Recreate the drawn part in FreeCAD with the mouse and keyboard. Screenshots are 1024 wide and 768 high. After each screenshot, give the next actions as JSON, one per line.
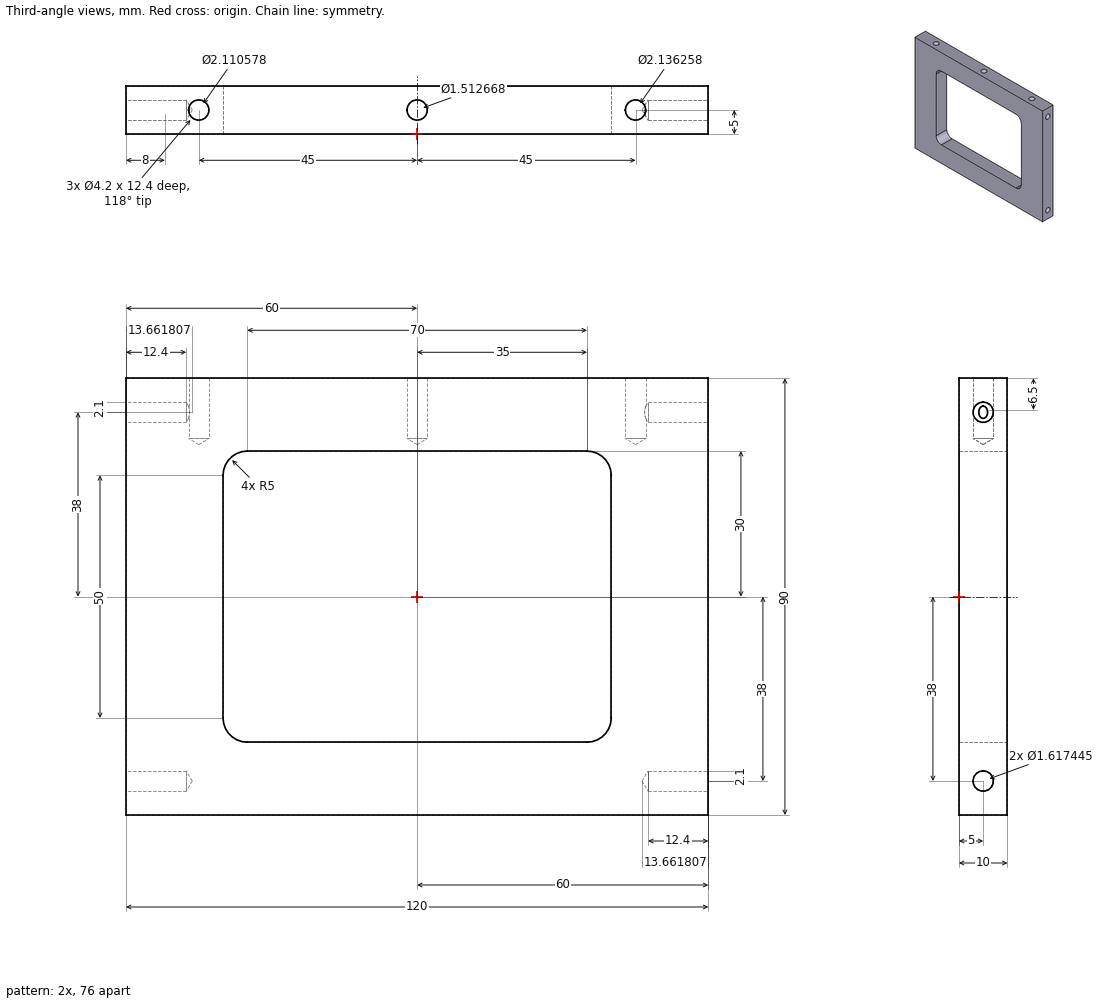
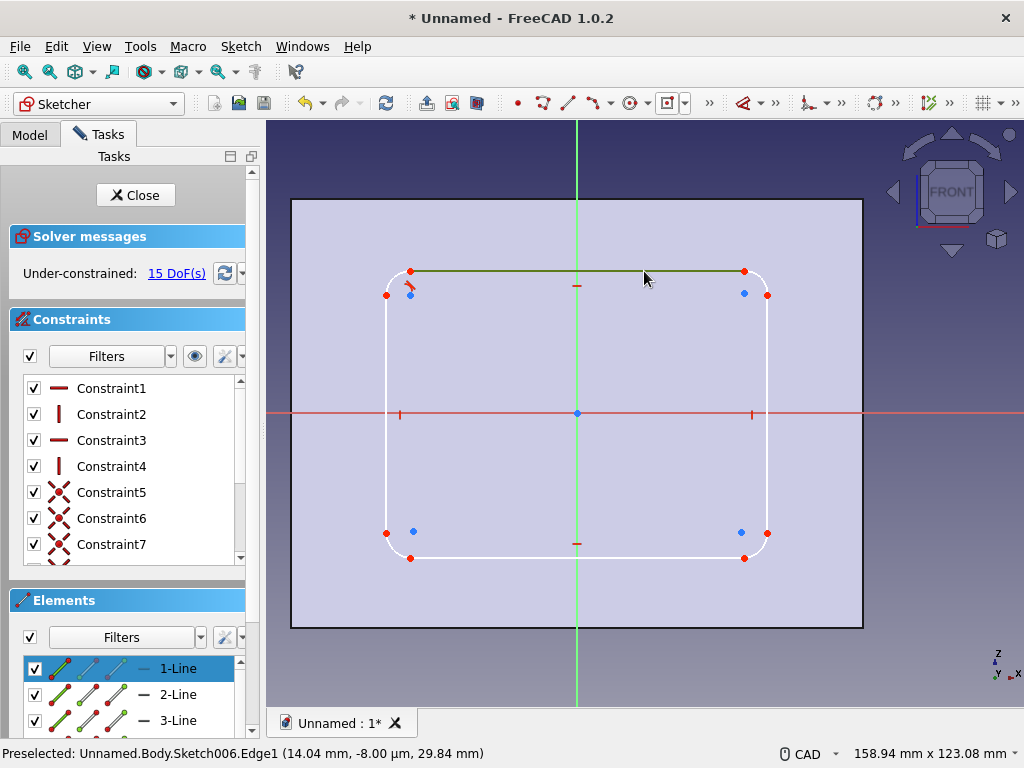
{"action": "left_click", "coordinate": [765, 284]}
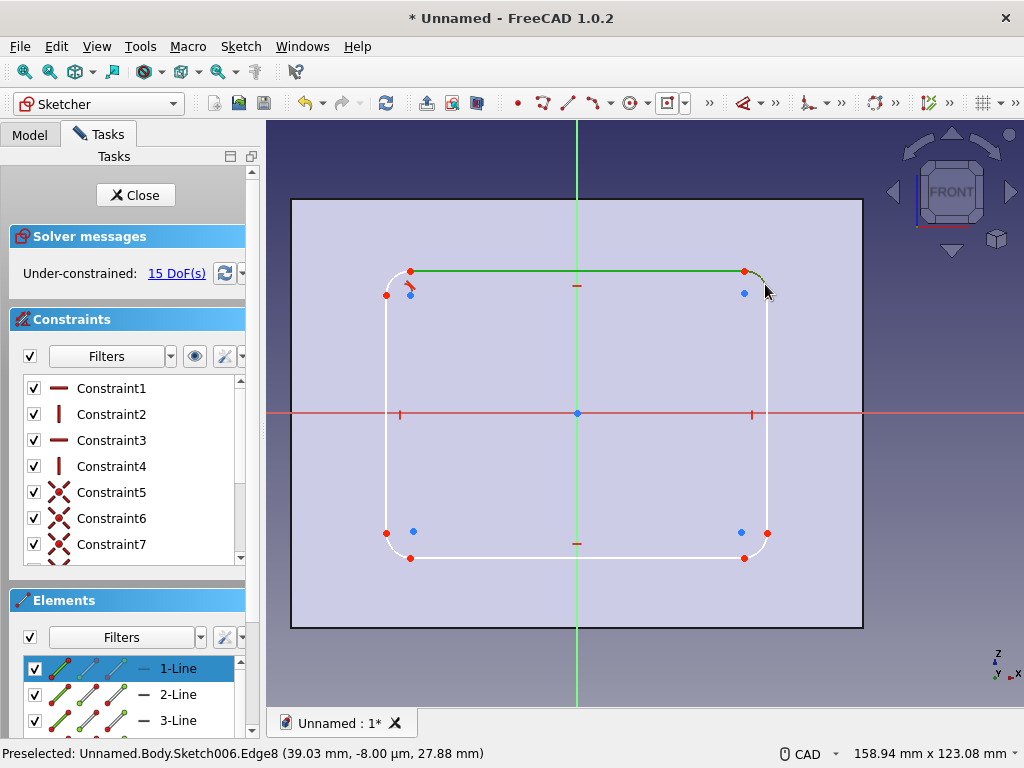
{"action": "key", "text": "t"}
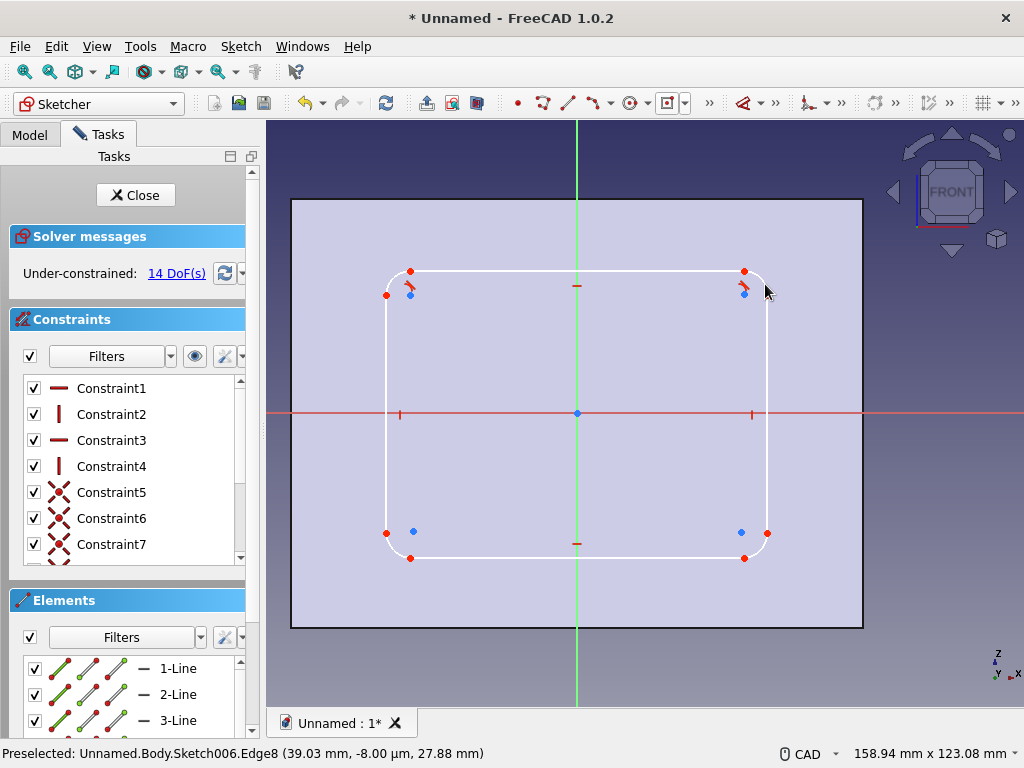
{"action": "left_click", "coordinate": [386, 367]}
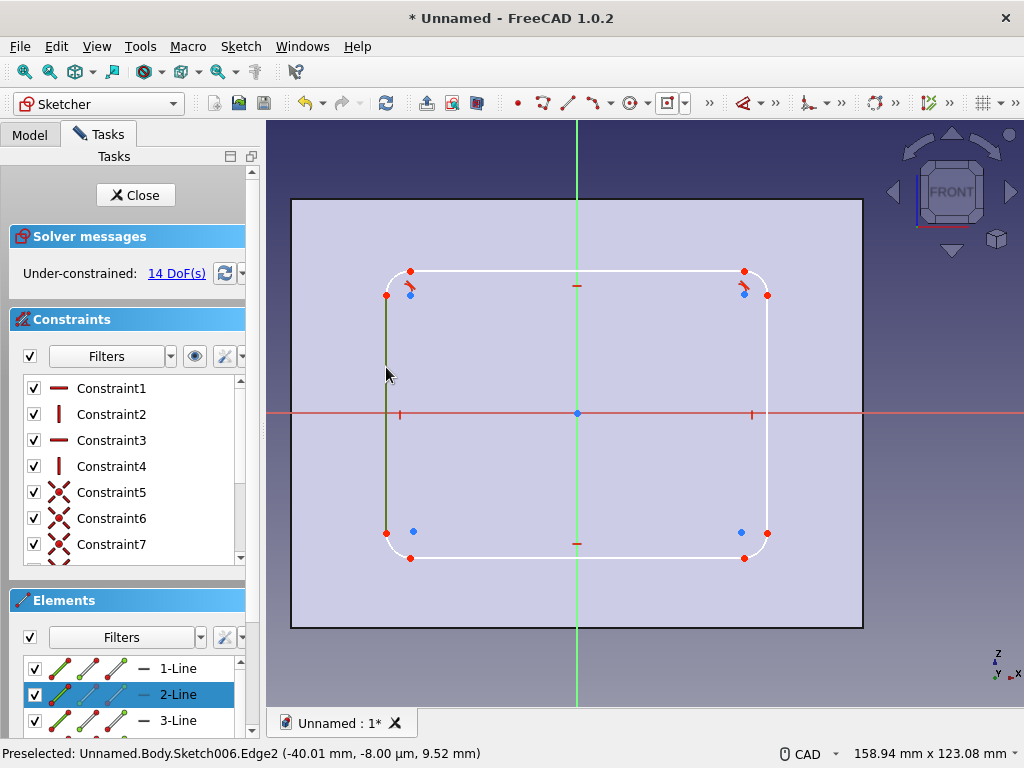
{"action": "left_click", "coordinate": [400, 274]}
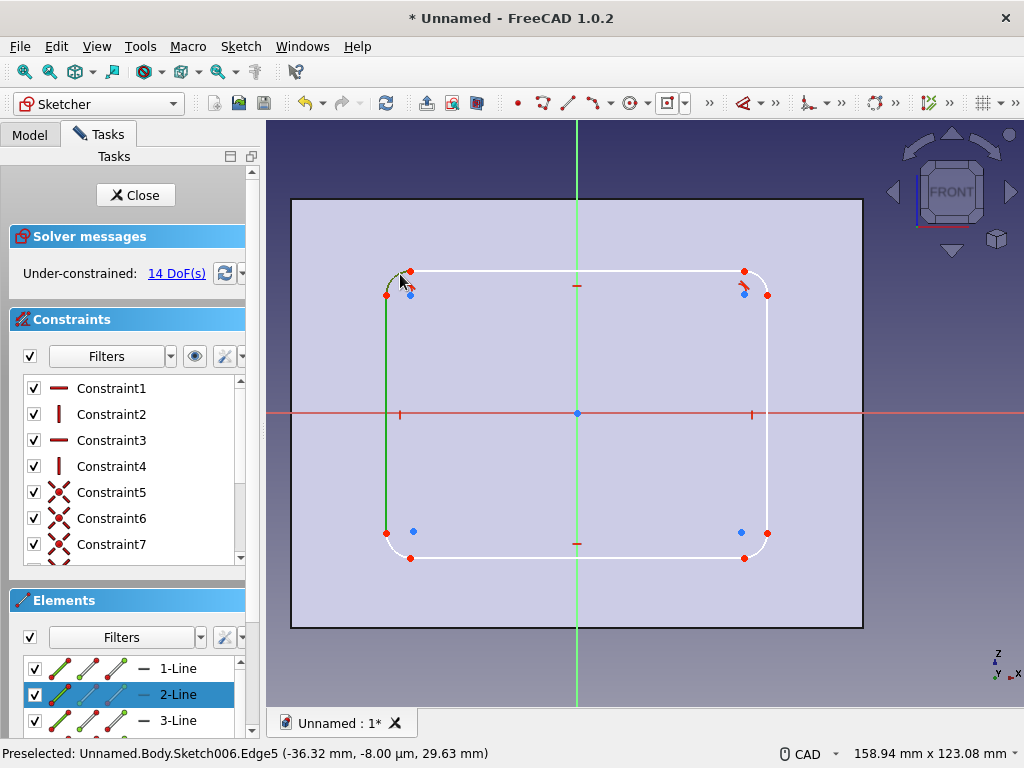
{"action": "key", "text": "t"}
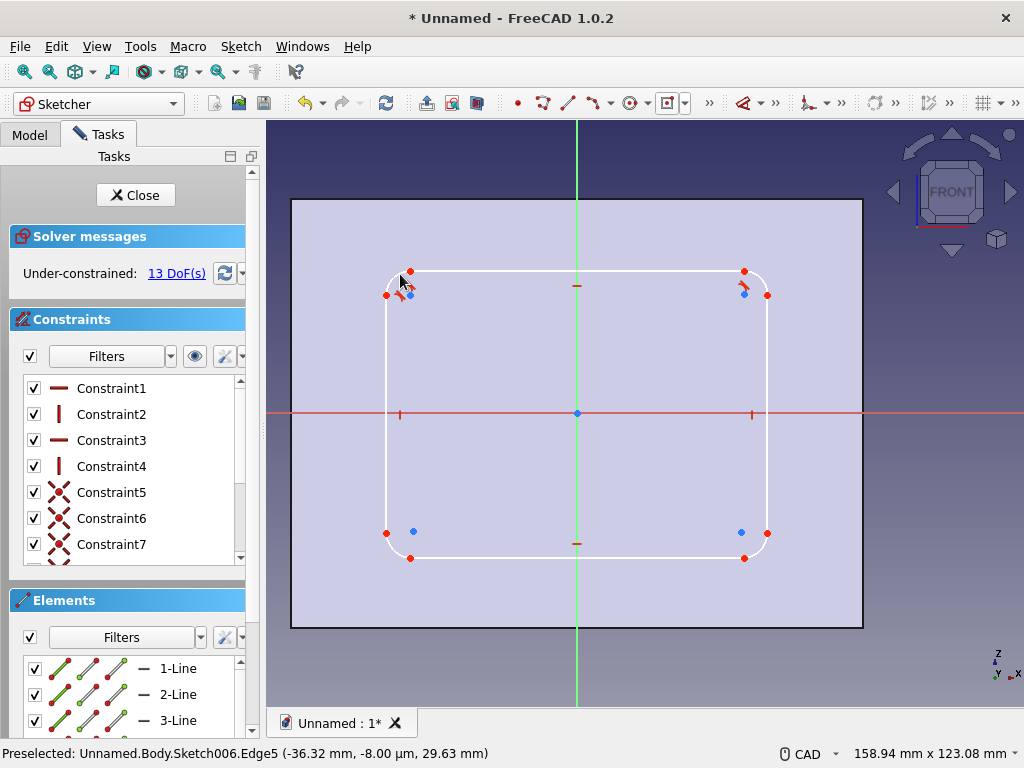
{"action": "left_click", "coordinate": [386, 367]}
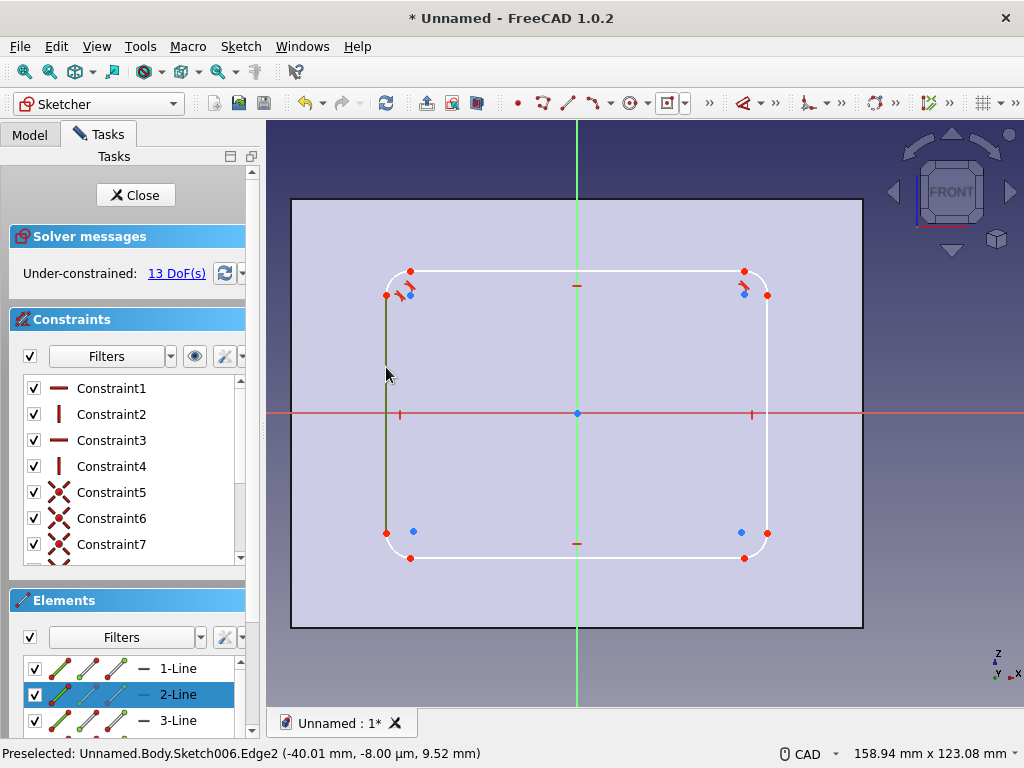
{"action": "scroll", "coordinate": [390, 544], "scroll_direction": "up", "scroll_amount": 2}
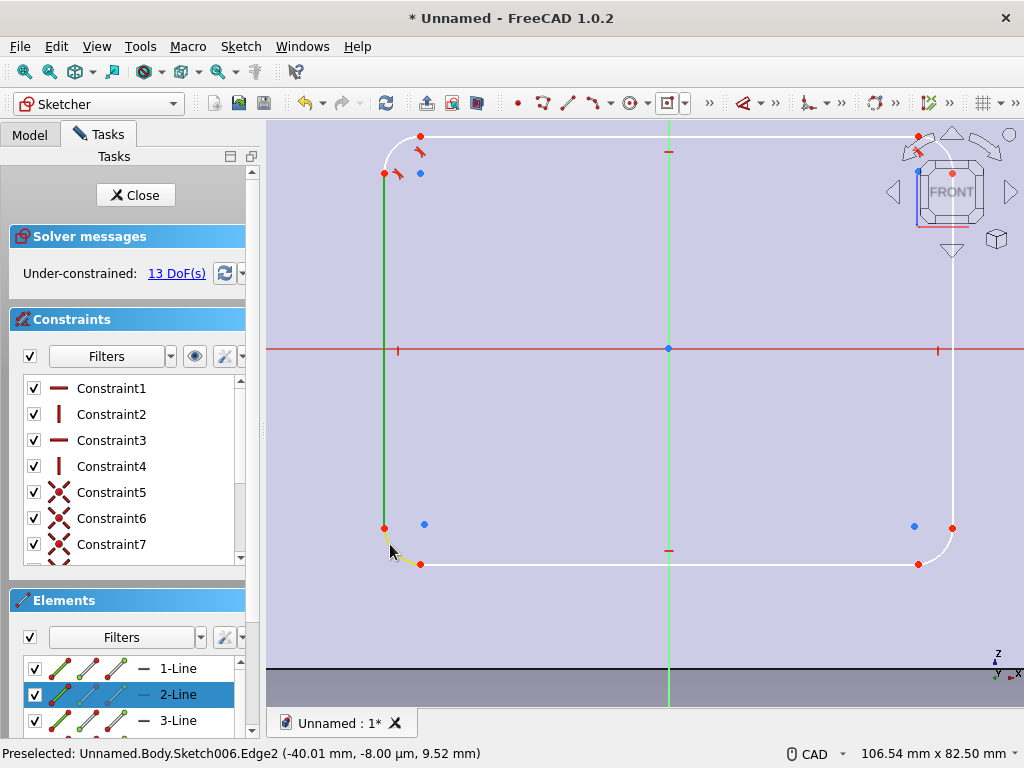
{"action": "left_click", "coordinate": [389, 544]}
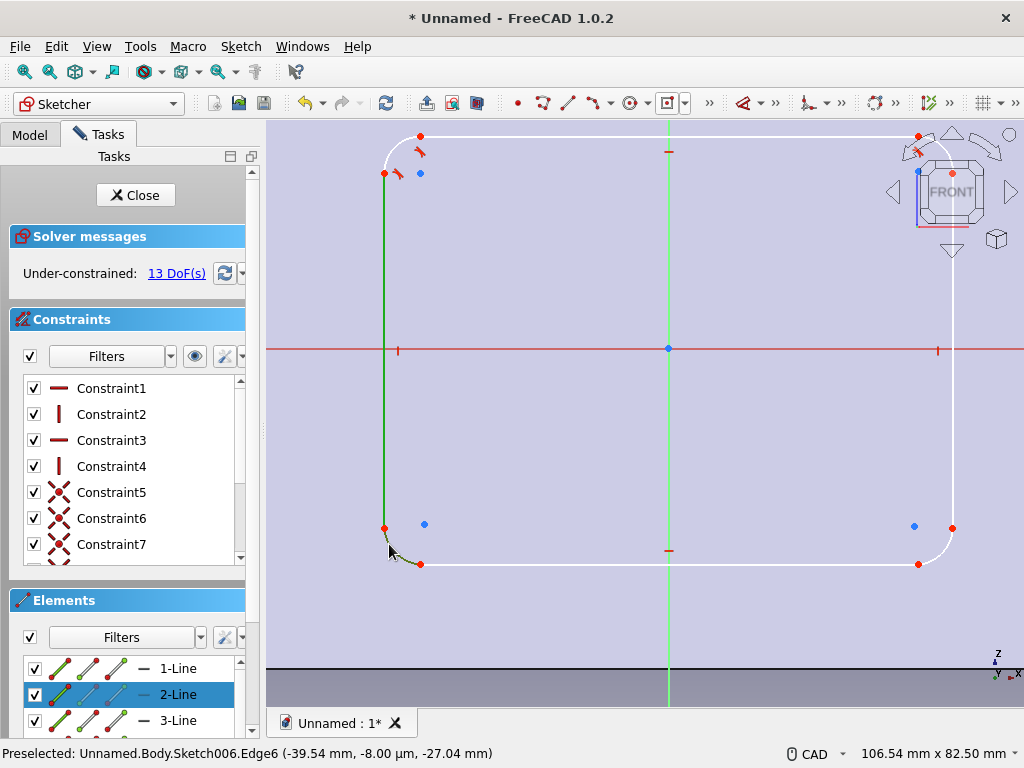
{"action": "key", "text": "t"}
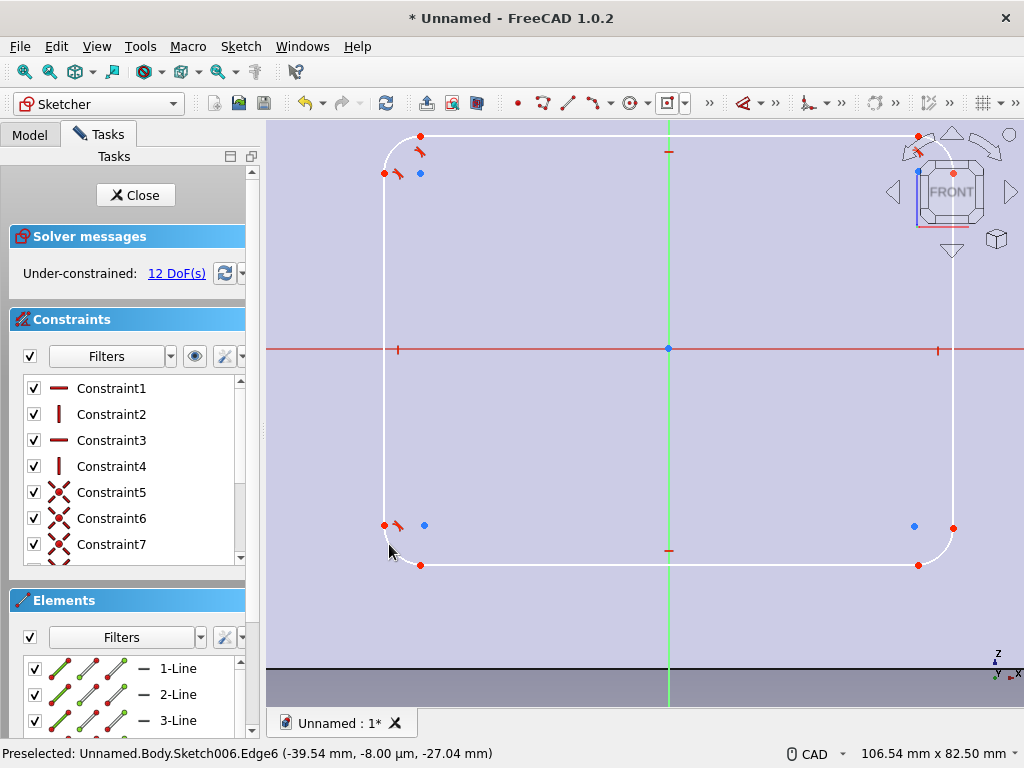
{"action": "left_click", "coordinate": [570, 565]}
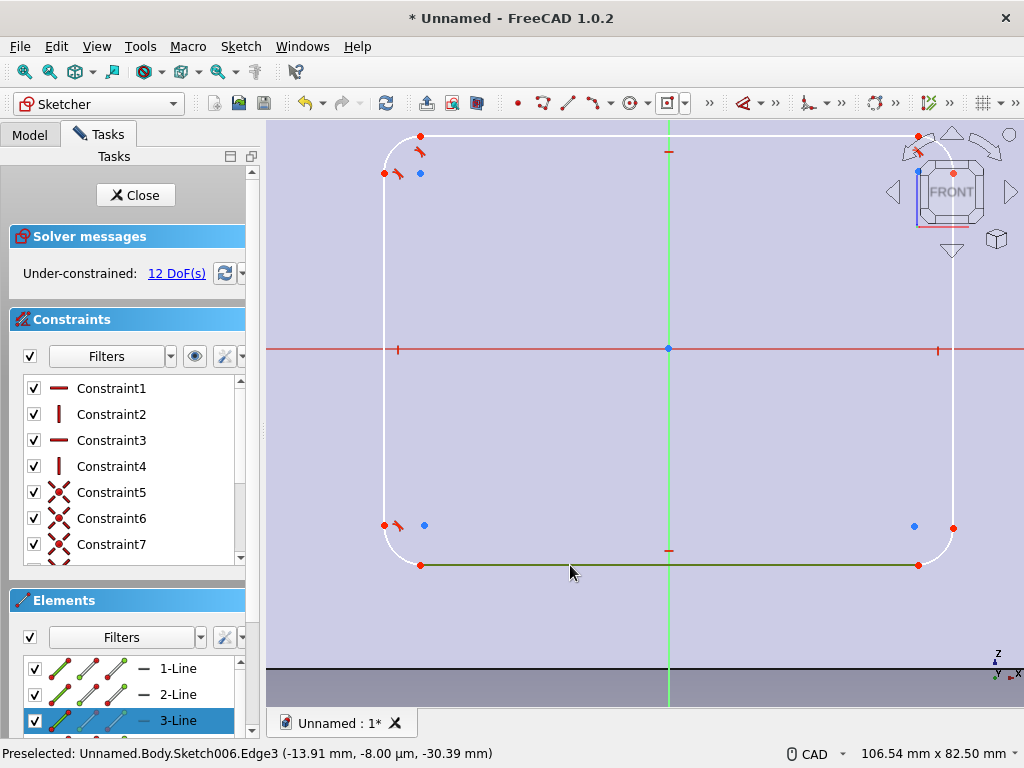
{"action": "left_click", "coordinate": [388, 542]}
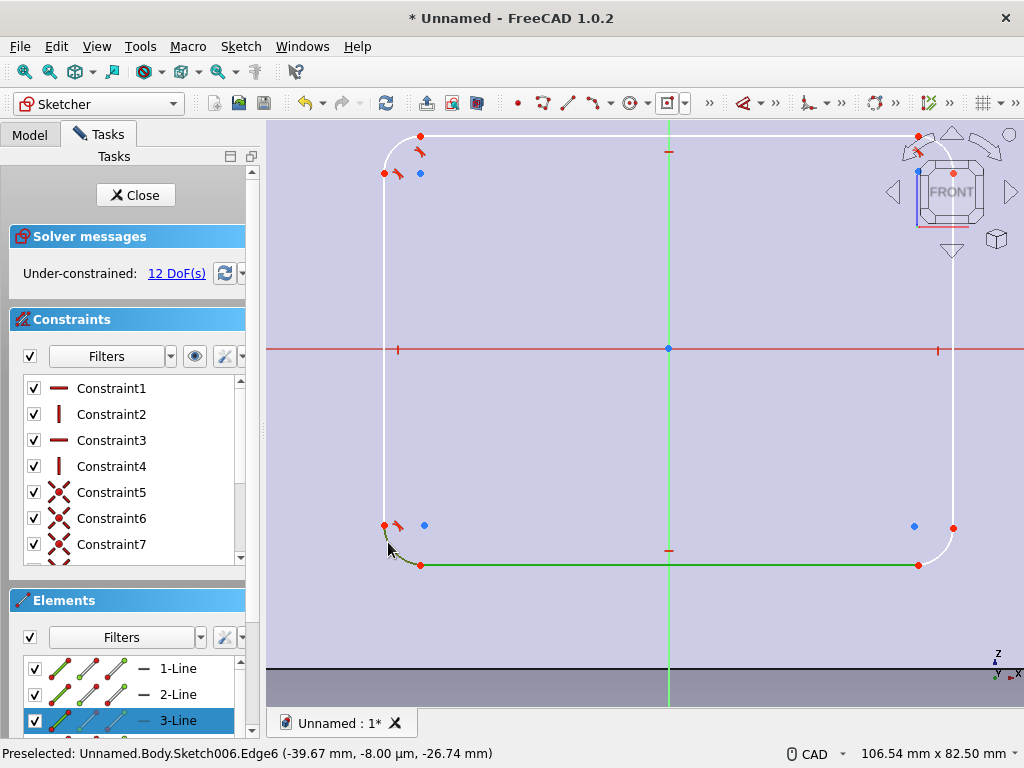
{"action": "key", "text": "t"}